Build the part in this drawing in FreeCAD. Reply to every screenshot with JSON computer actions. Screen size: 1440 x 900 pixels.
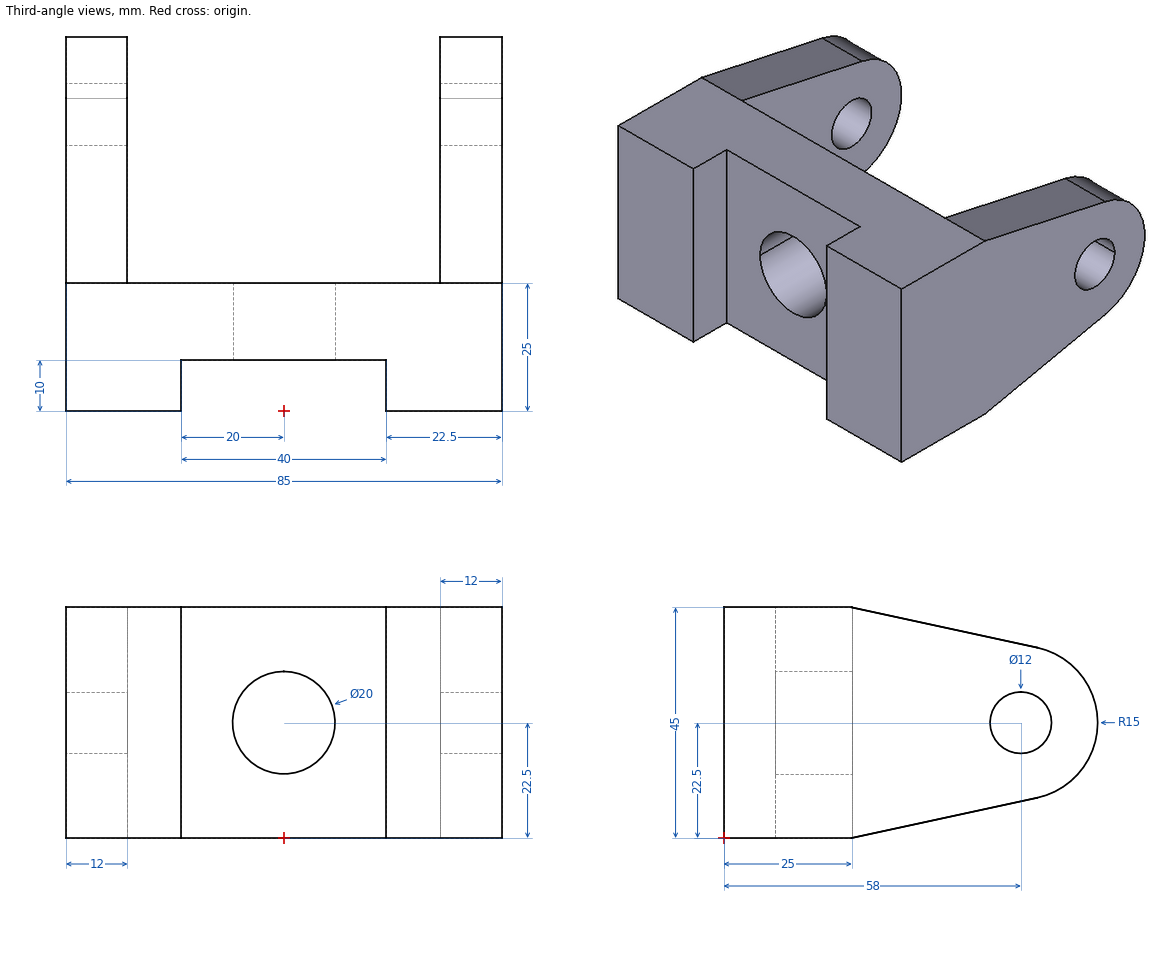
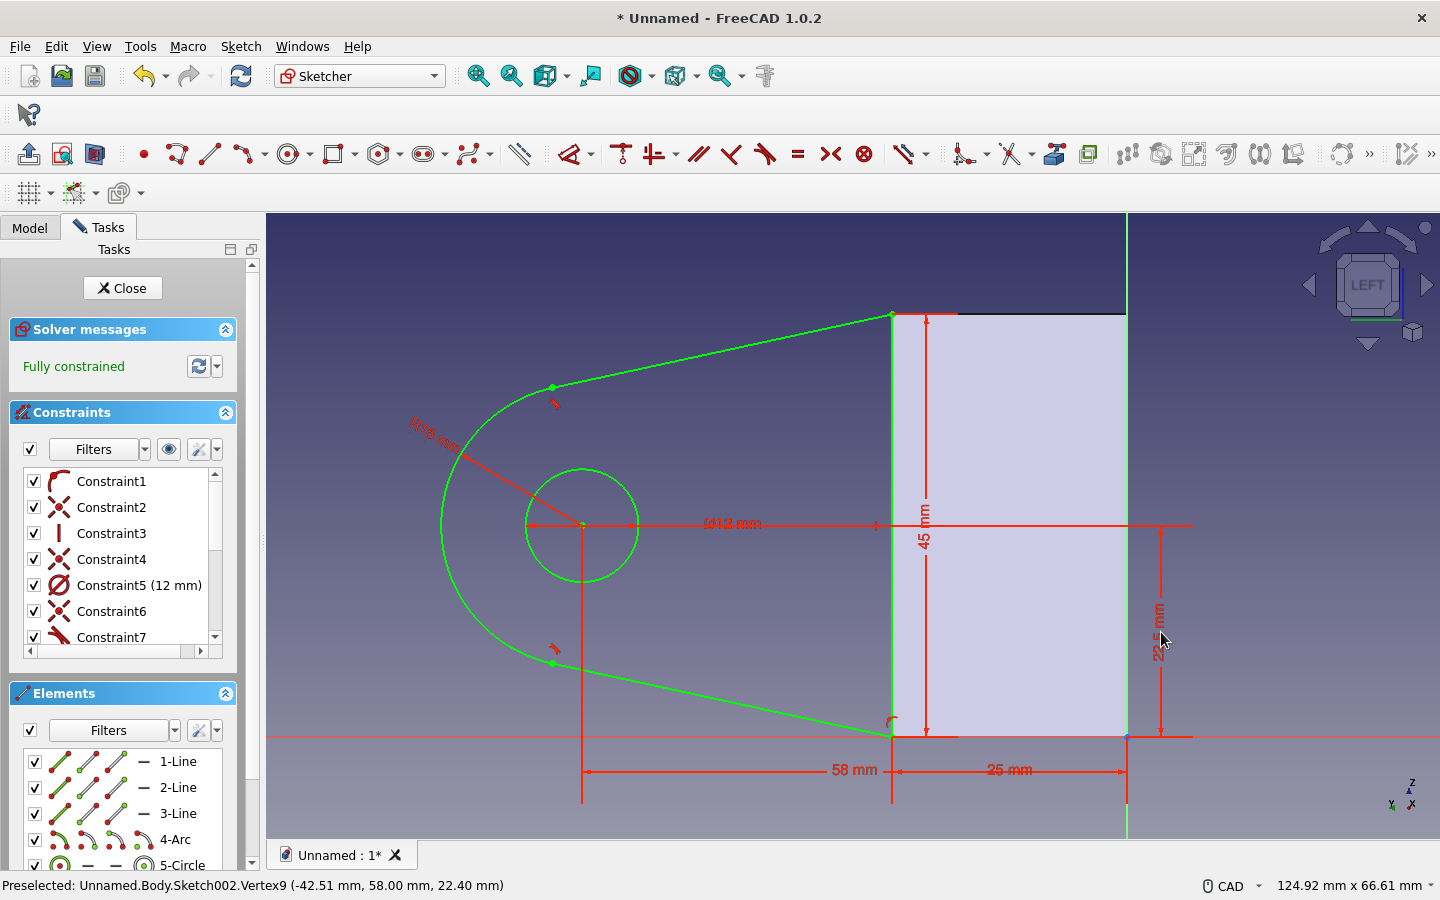
{"action": "left_click", "coordinate": [123, 288]}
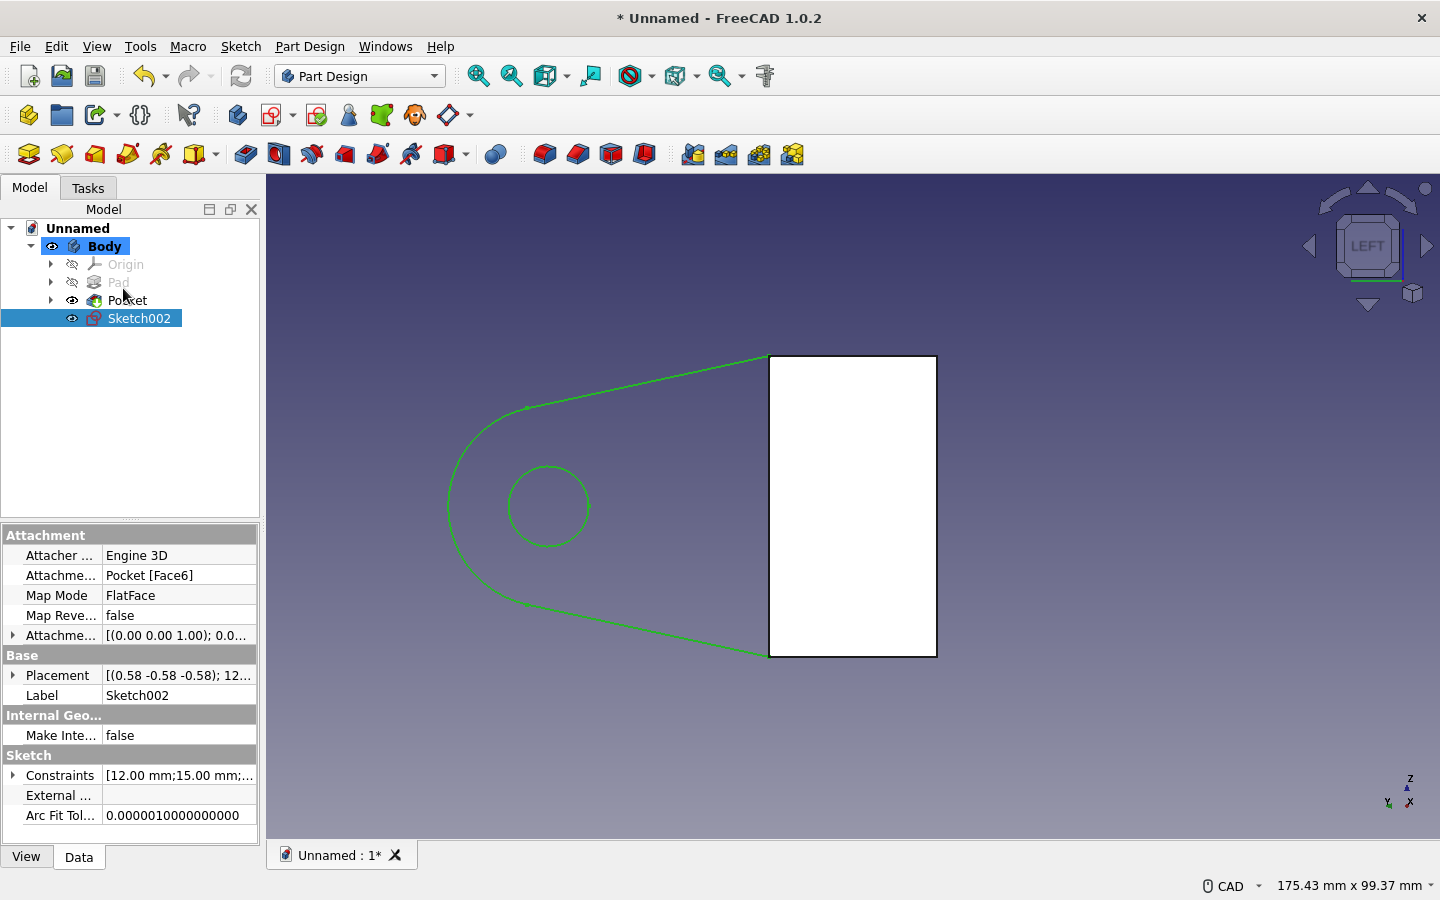
{"action": "left_click", "coordinate": [29, 154]}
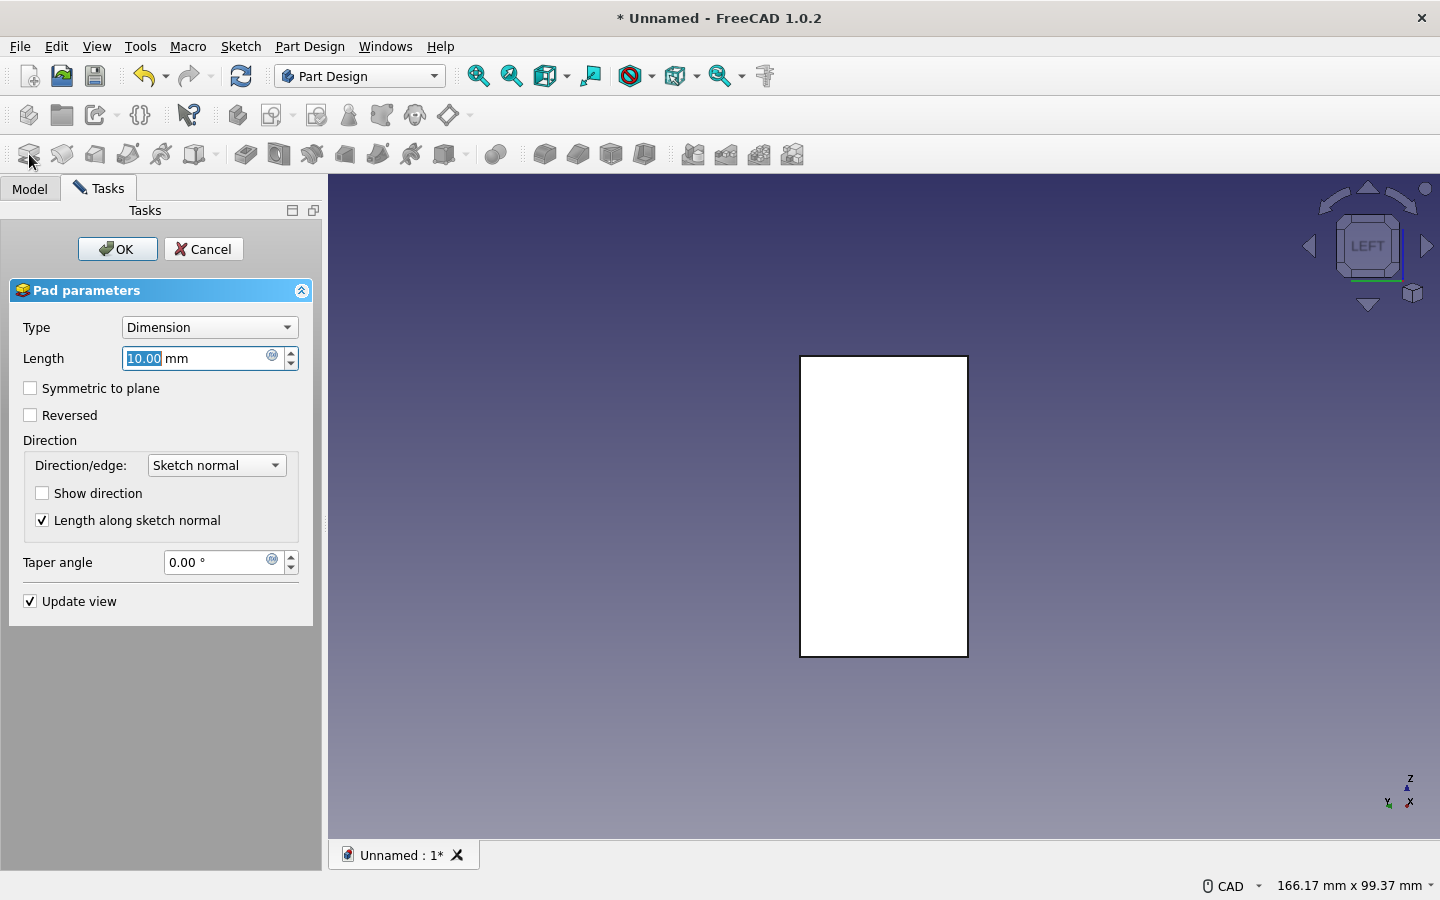
{"action": "type", "text": "12"}
{"action": "key", "text": "Tab"}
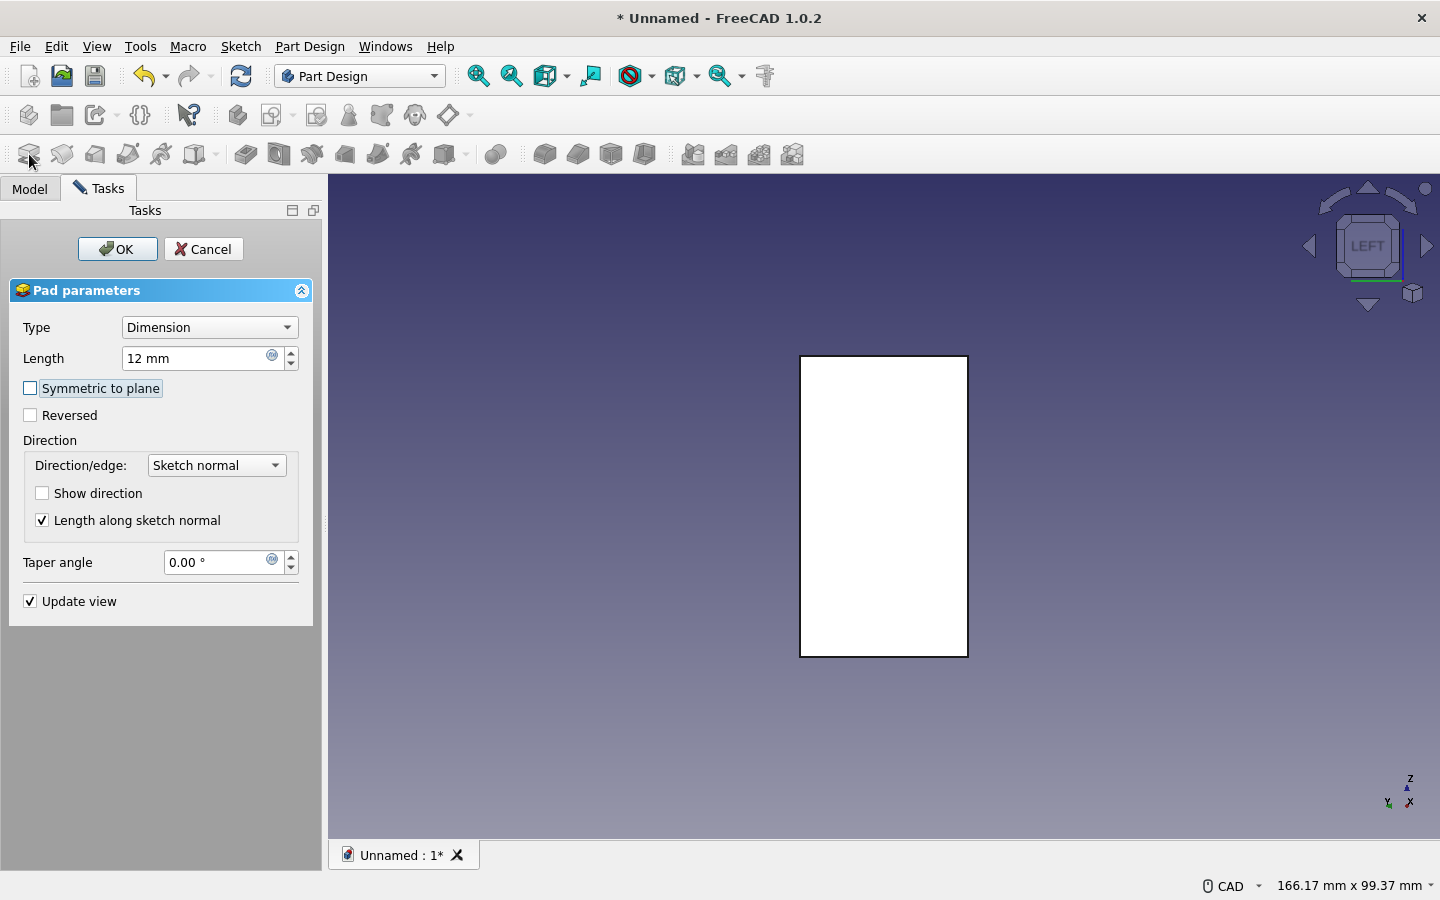
{"action": "left_click", "coordinate": [31, 415]}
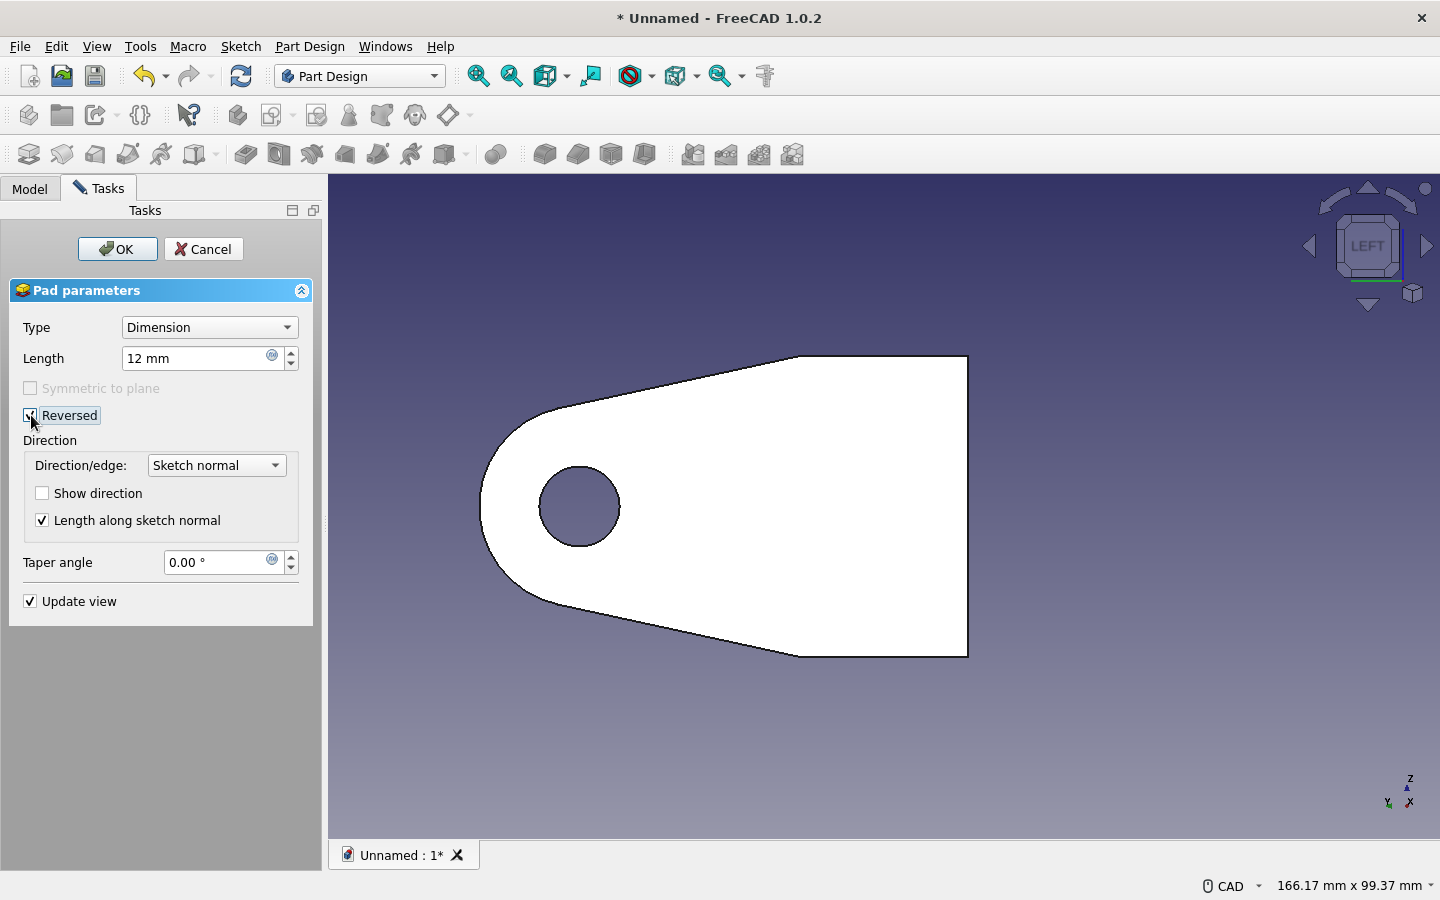
{"action": "left_click", "coordinate": [118, 249]}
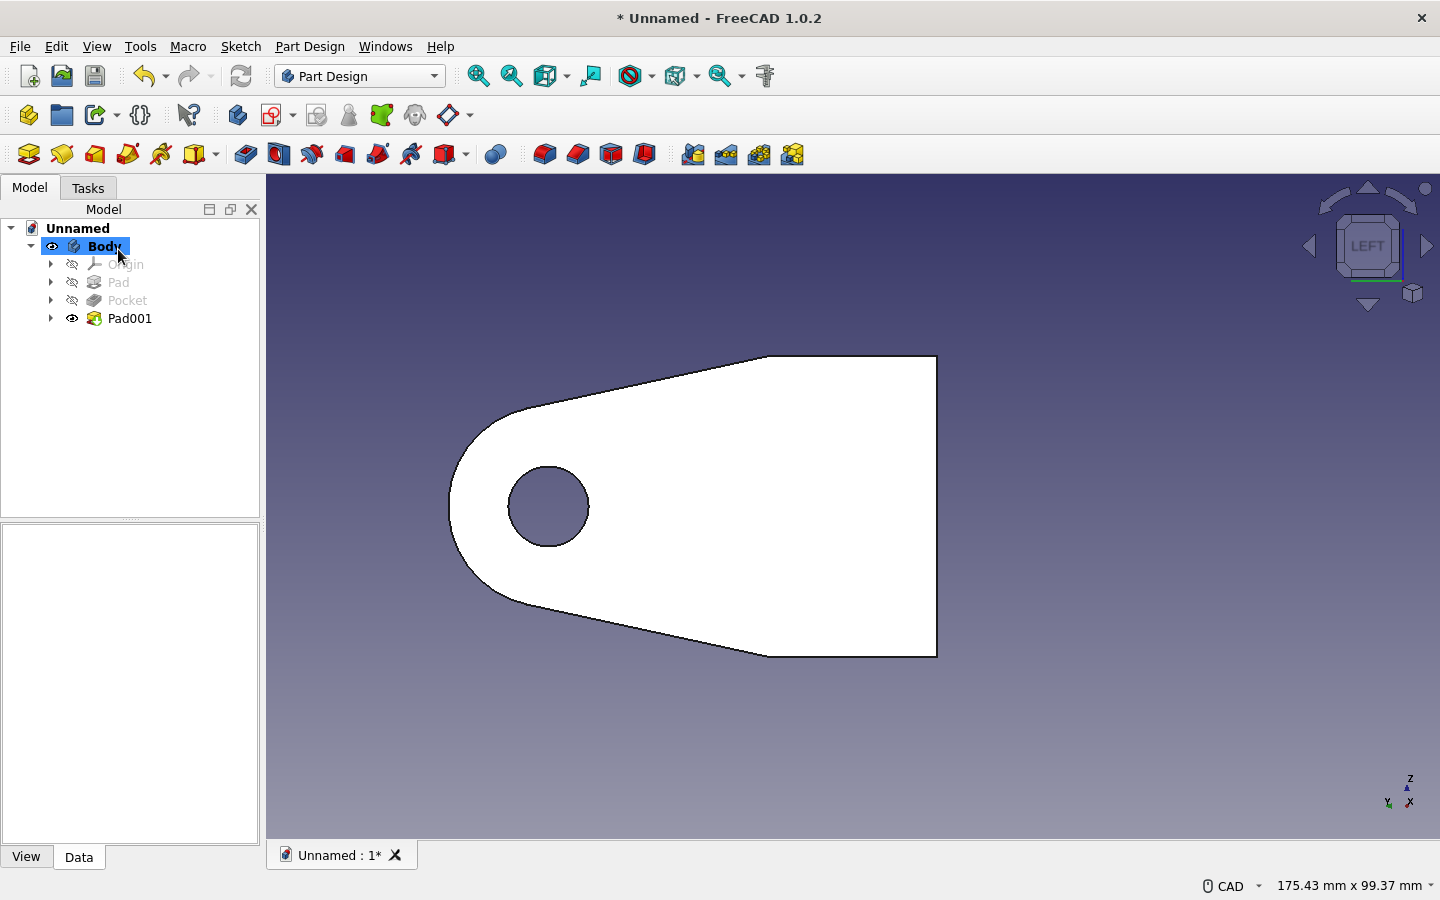
{"action": "left_click", "coordinate": [51, 264]}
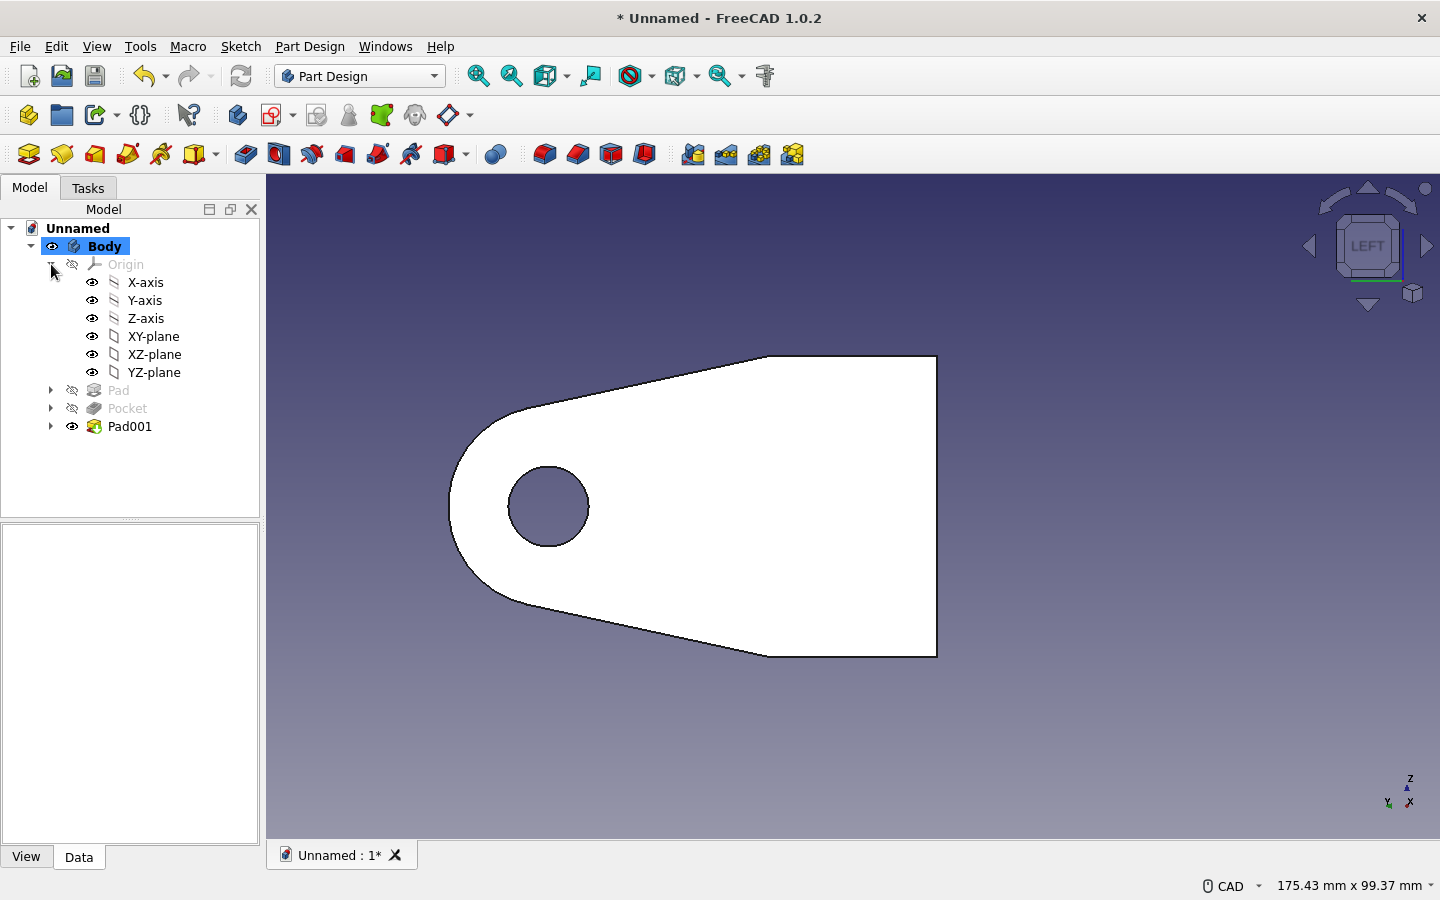
{"action": "left_click", "coordinate": [137, 372]}